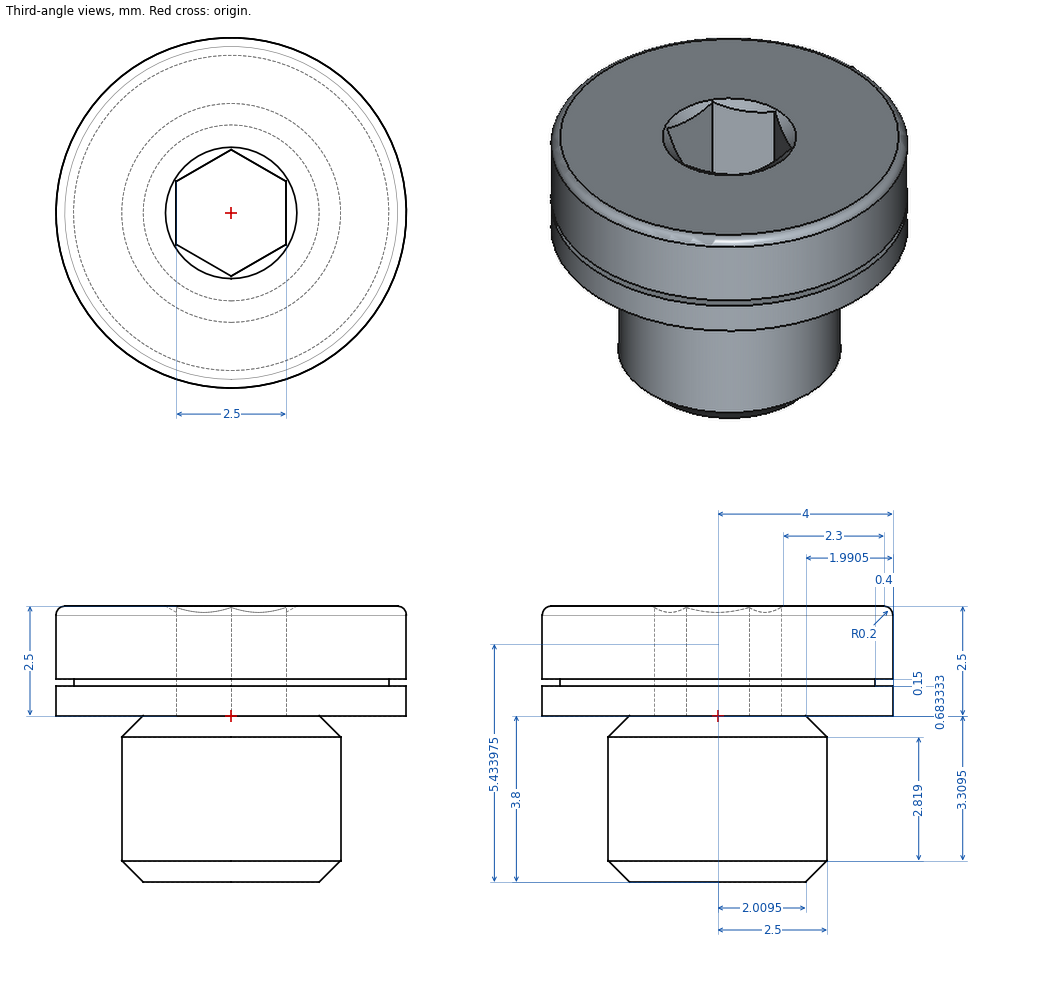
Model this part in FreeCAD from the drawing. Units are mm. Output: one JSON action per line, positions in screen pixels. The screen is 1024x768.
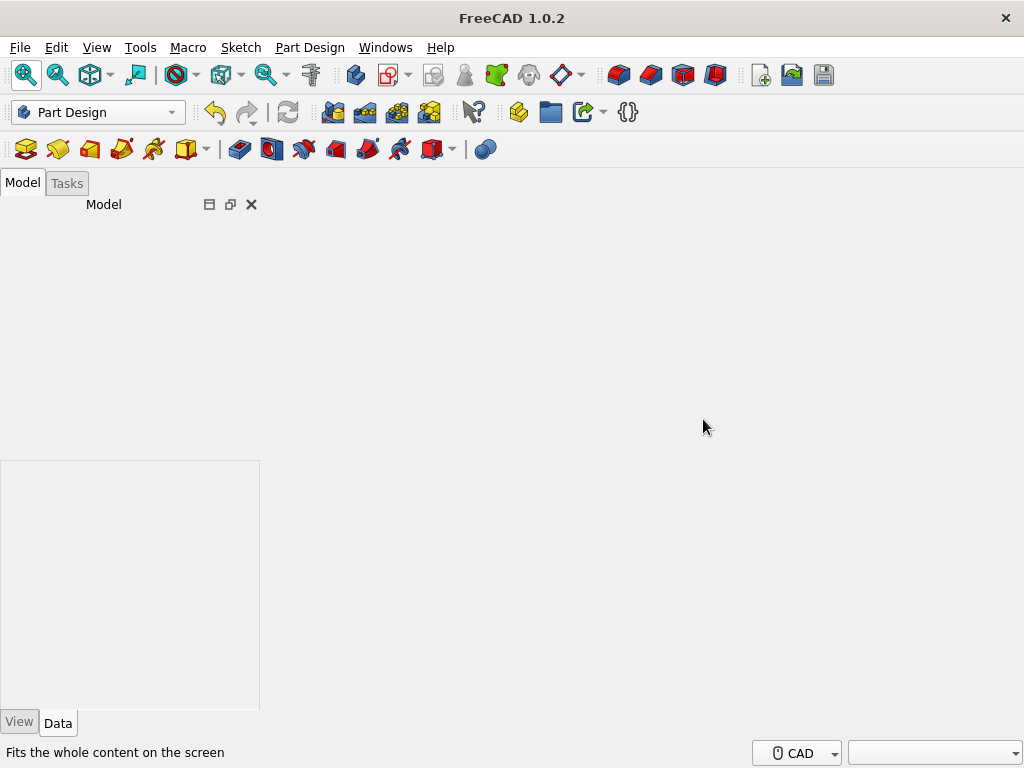
{"action": "key", "text": "ctrl+n"}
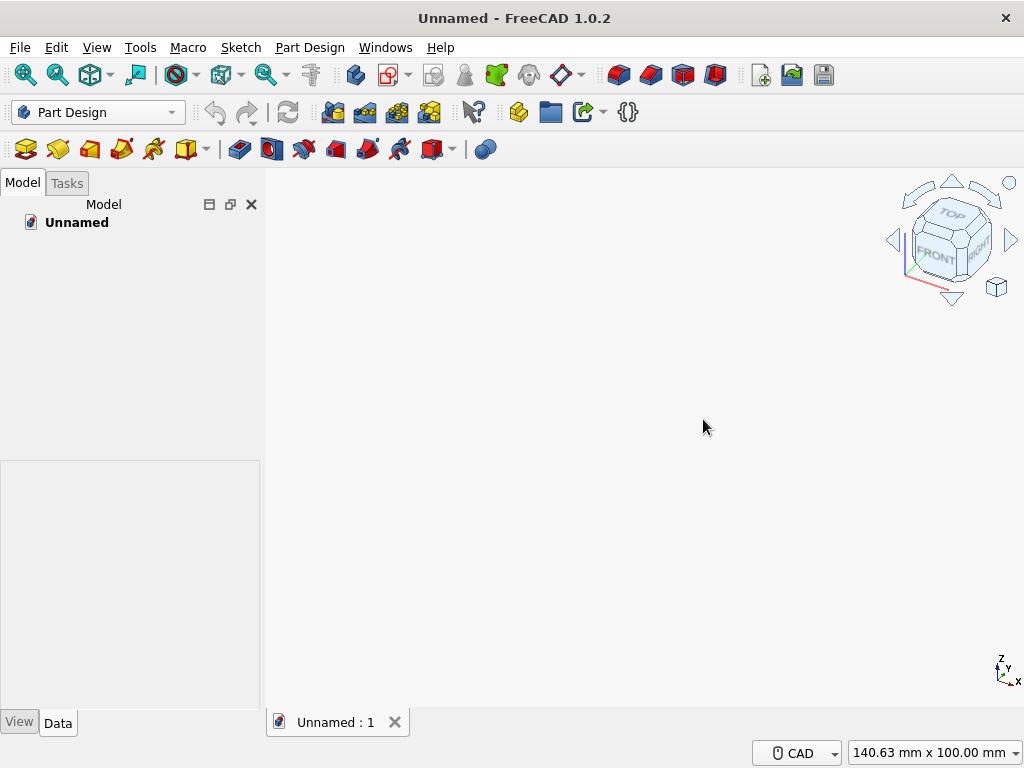
{"action": "left_click", "coordinate": [388, 76]}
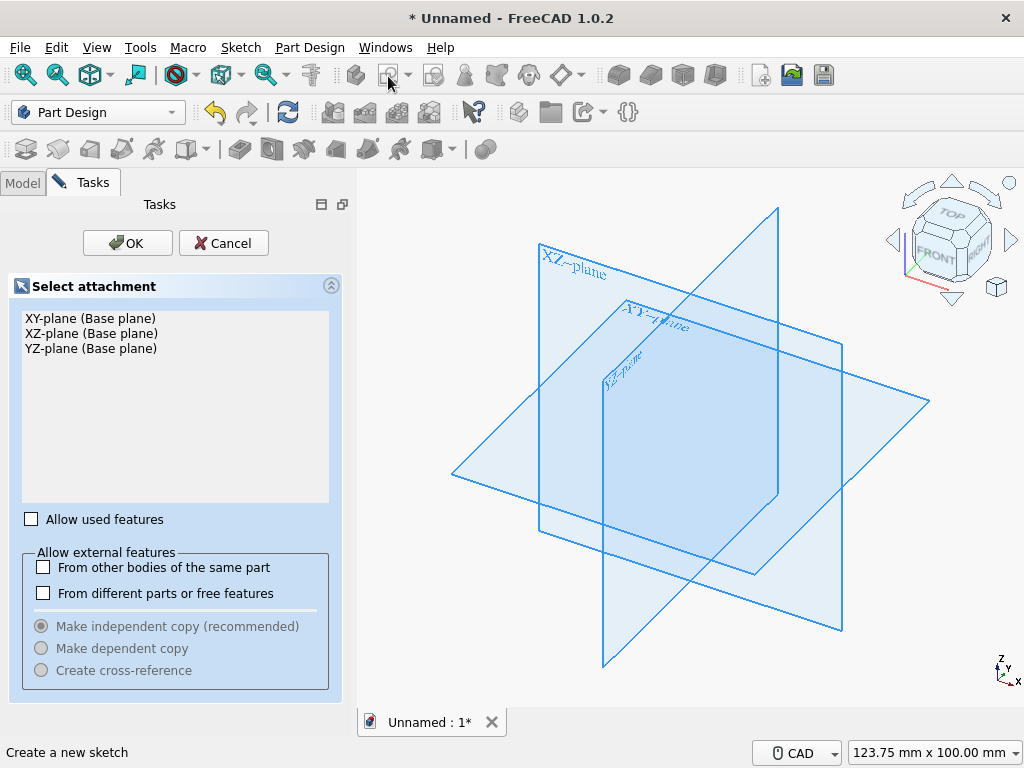
{"action": "left_click", "coordinate": [82, 348]}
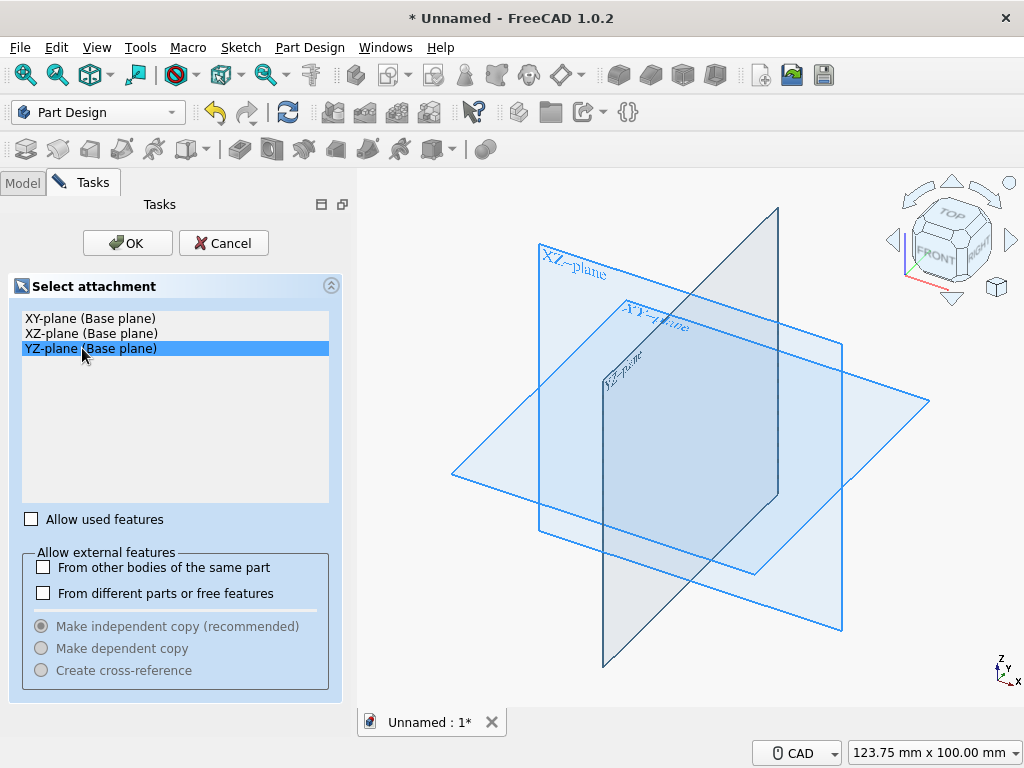
{"action": "left_click", "coordinate": [128, 243]}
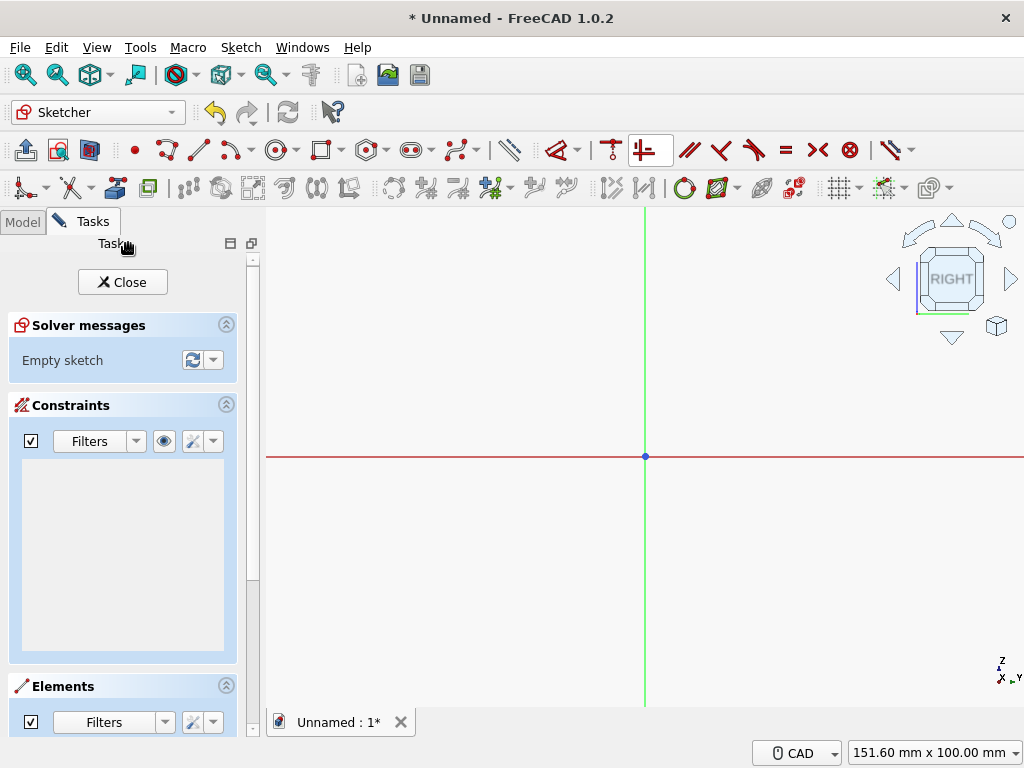
{"action": "scroll", "coordinate": [665, 461], "scroll_direction": "up", "scroll_amount": 11}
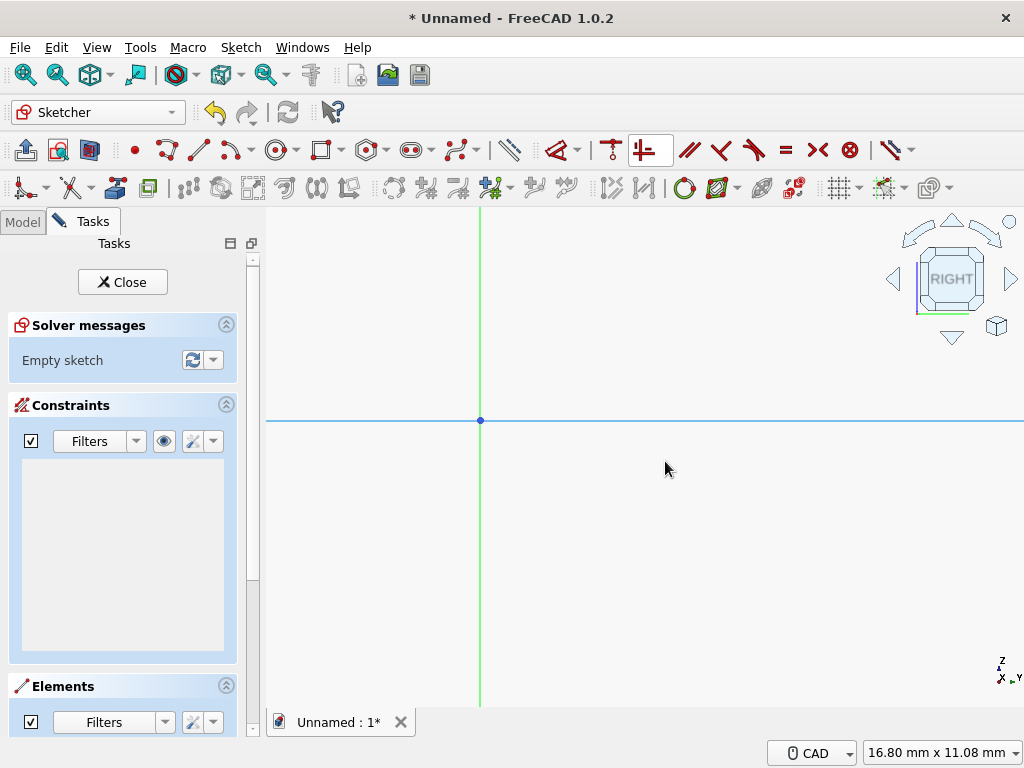
{"action": "key", "text": "g m"}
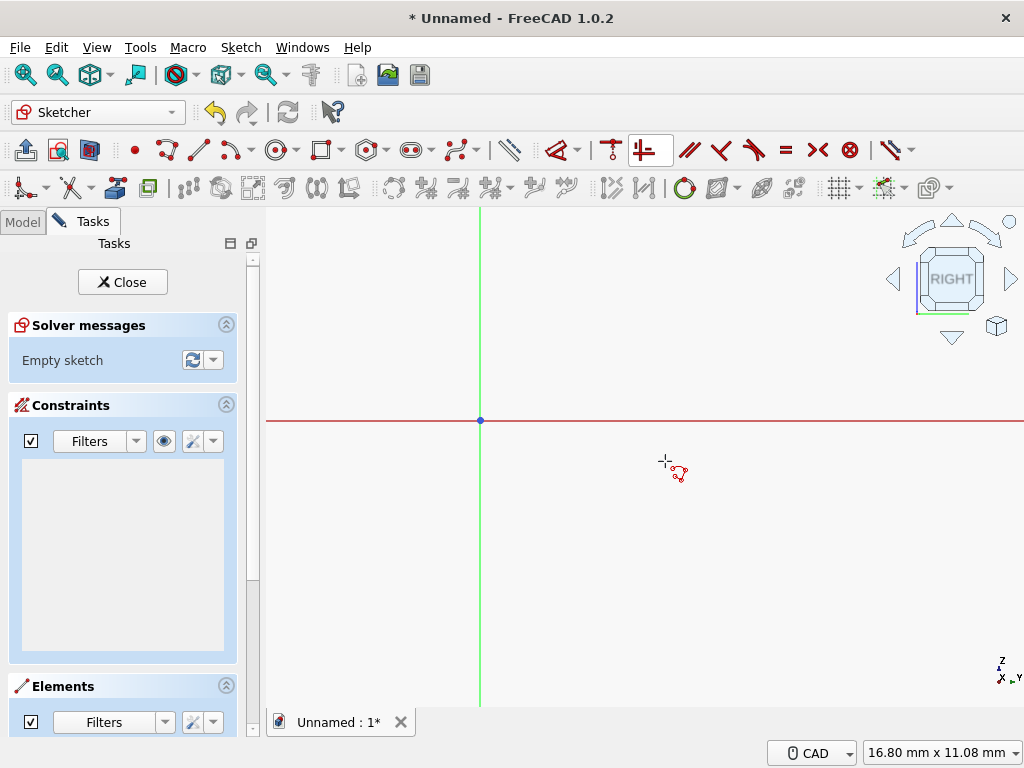
{"action": "left_click", "coordinate": [652, 308]}
{"action": "left_click", "coordinate": [548, 308]}
{"action": "left_click", "coordinate": [480, 347]}
{"action": "left_click", "coordinate": [489, 592]}
{"action": "left_click", "coordinate": [571, 592]}
{"action": "left_click", "coordinate": [593, 570]}
{"action": "left_click", "coordinate": [593, 443]}
{"action": "left_click", "coordinate": [571, 421]}
{"action": "left_click", "coordinate": [661, 430]}
{"action": "left_click", "coordinate": [661, 390]}
{"action": "left_click", "coordinate": [643, 390]}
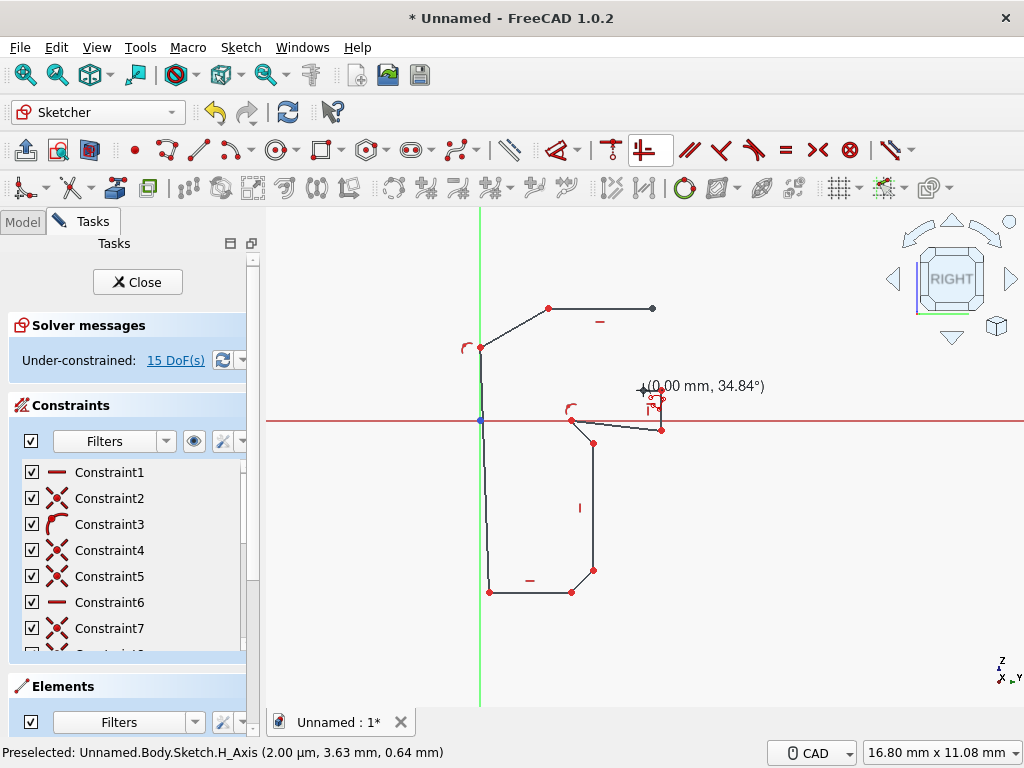
{"action": "scroll", "coordinate": [643, 383], "scroll_direction": "up", "scroll_amount": 5}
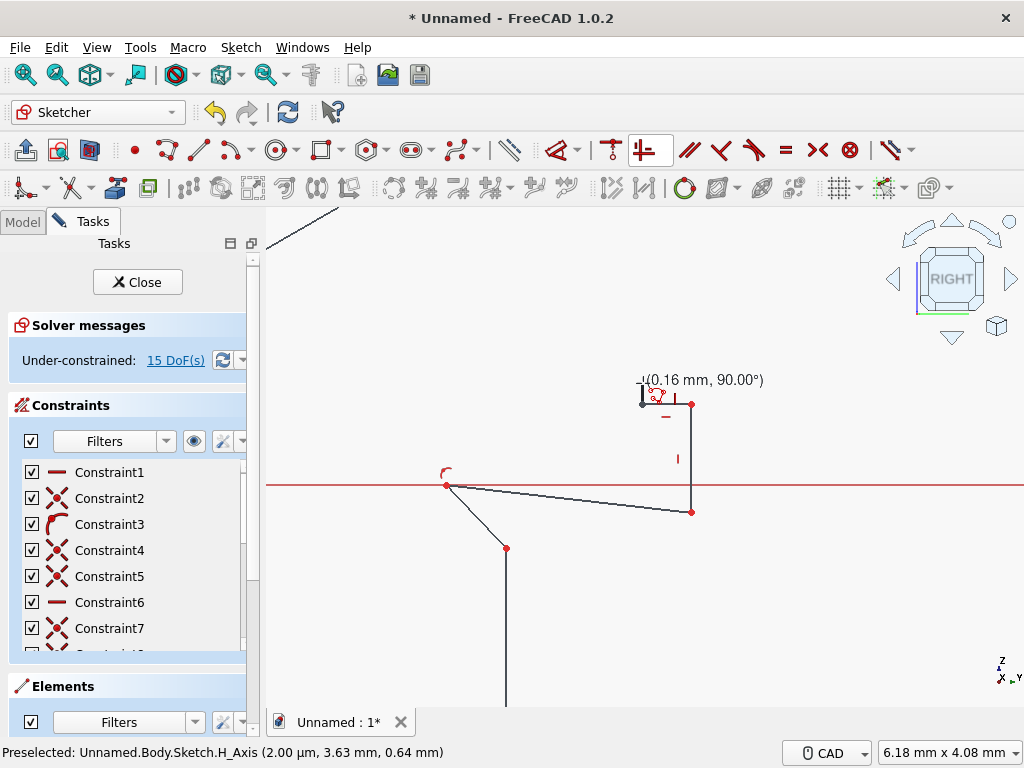
{"action": "left_click", "coordinate": [642, 383]}
{"action": "left_click", "coordinate": [690, 383]}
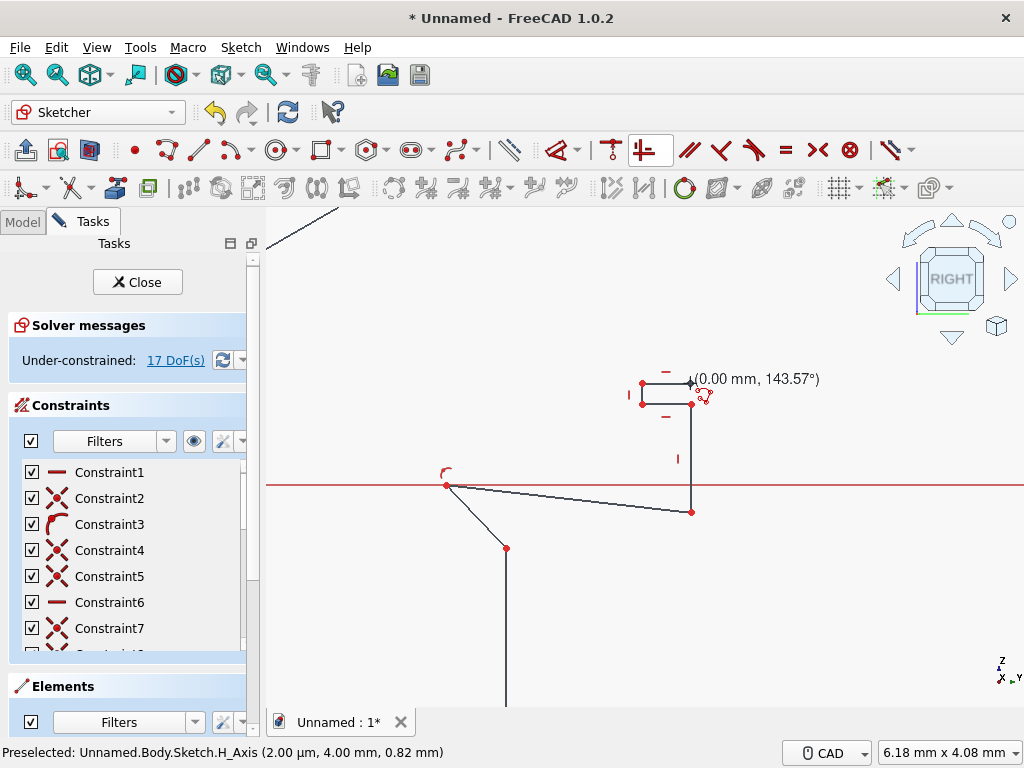
{"action": "scroll", "coordinate": [653, 394], "scroll_direction": "down", "scroll_amount": 5}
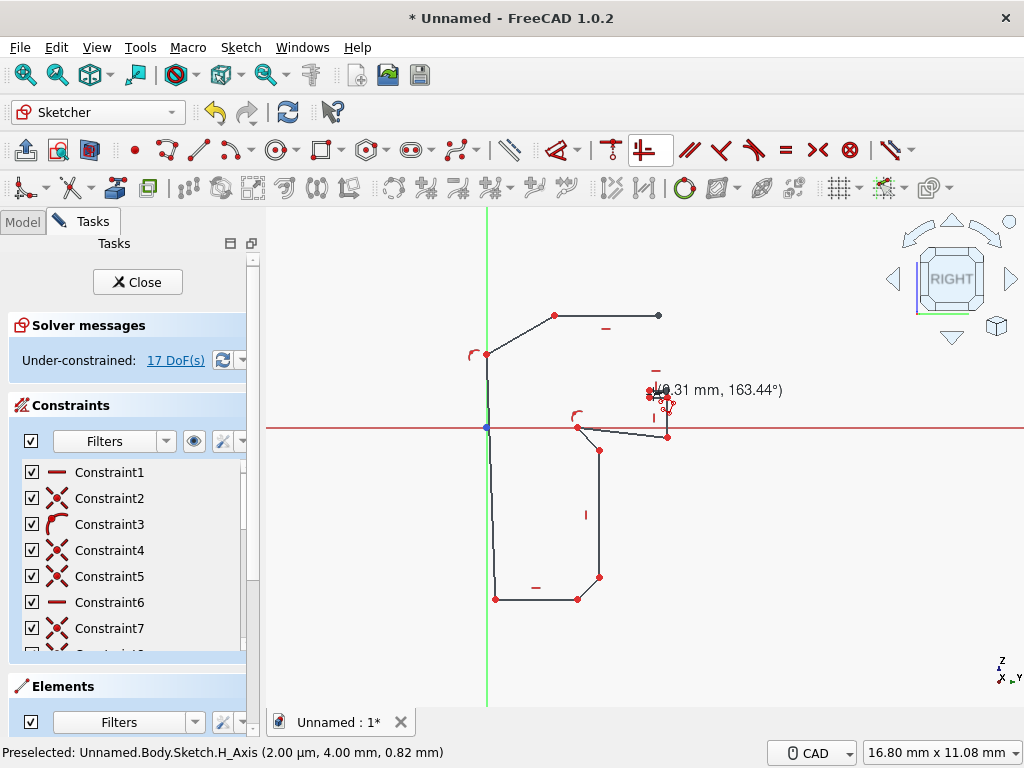
{"action": "scroll", "coordinate": [667, 324], "scroll_direction": "up", "scroll_amount": 2}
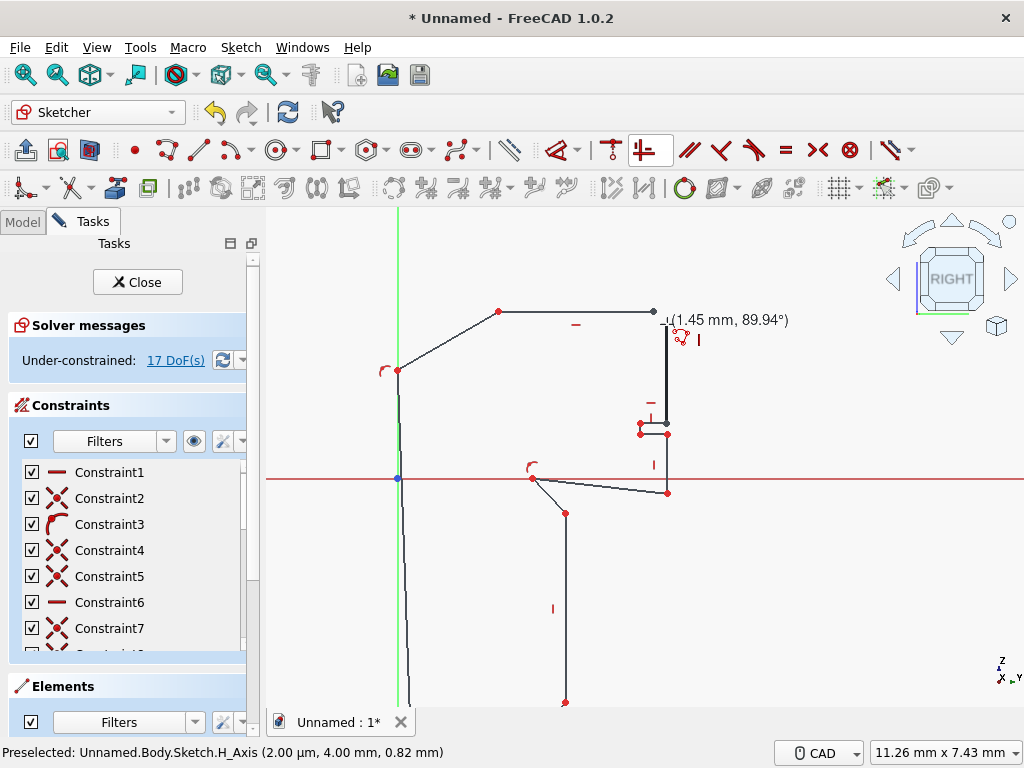
{"action": "left_click", "coordinate": [667, 324]}
{"action": "right_click", "coordinate": [667, 324]}